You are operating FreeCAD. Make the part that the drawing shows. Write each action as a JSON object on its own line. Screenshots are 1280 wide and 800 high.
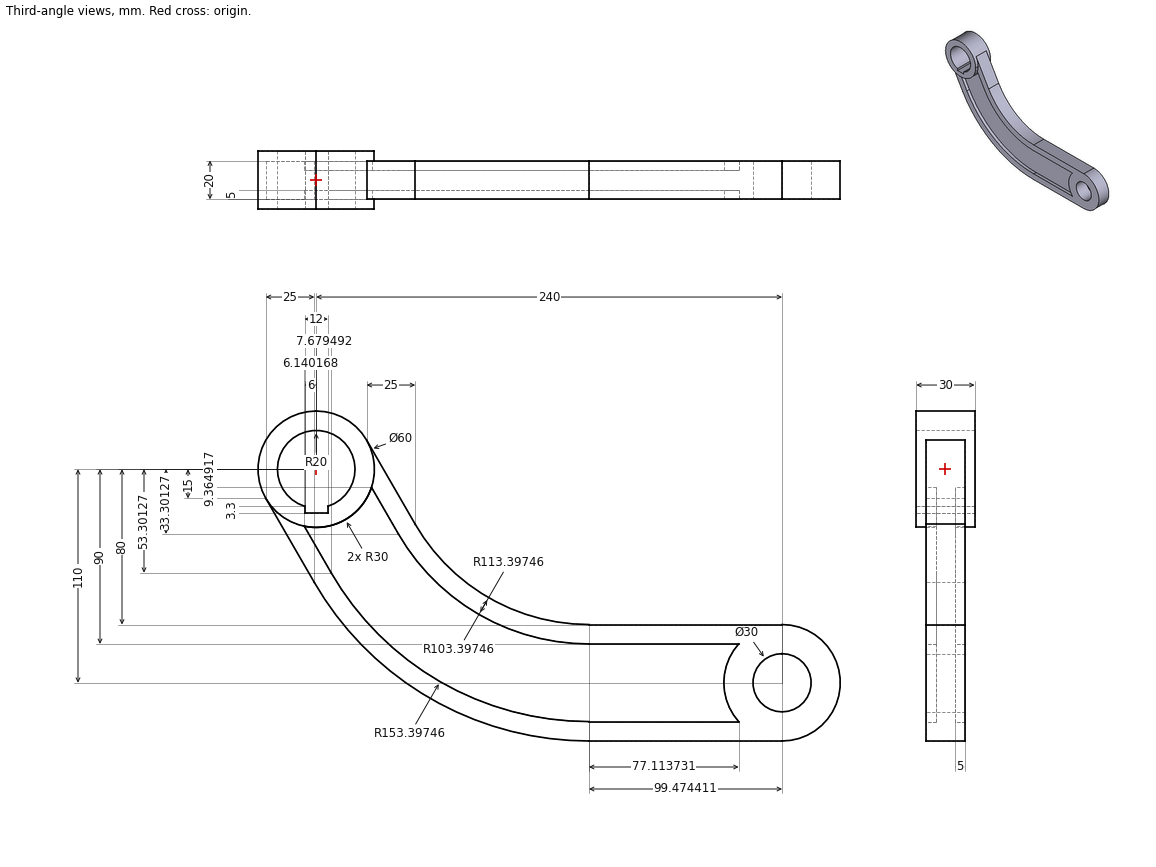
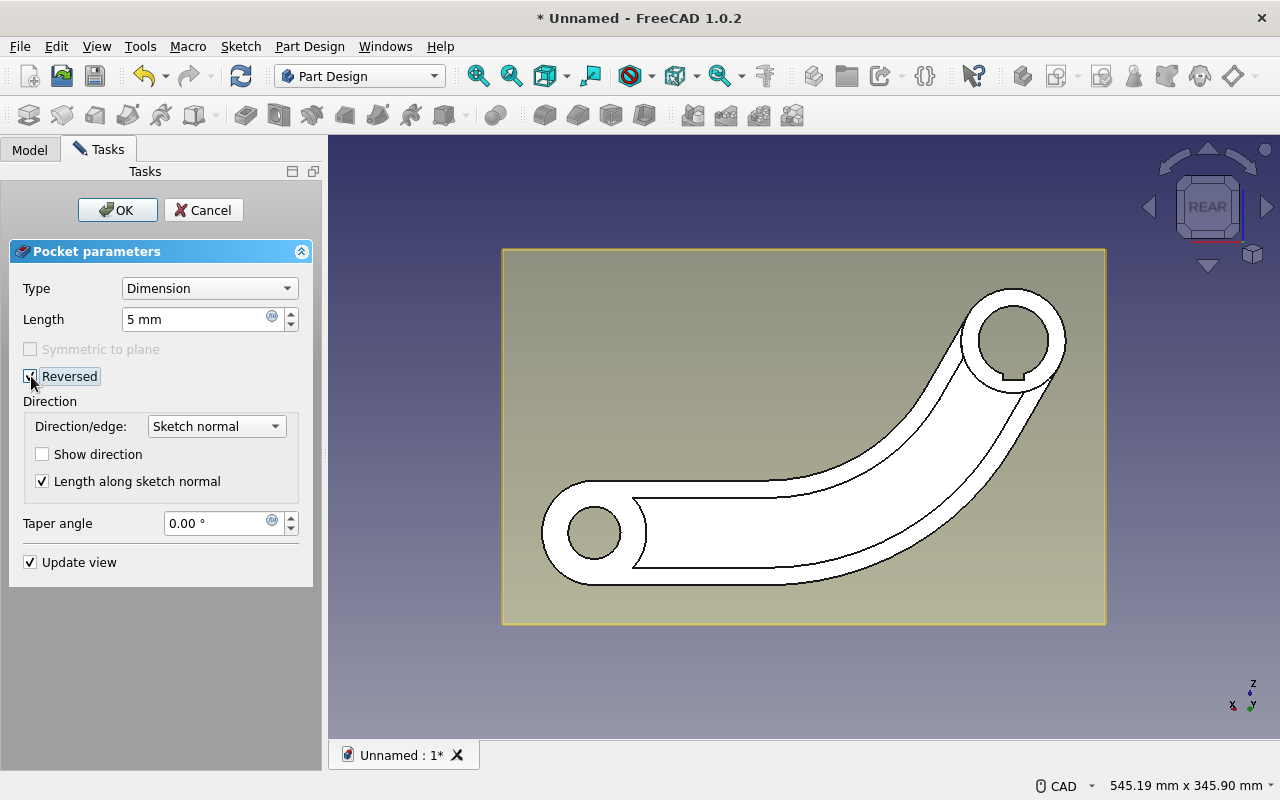
{"action": "left_click", "coordinate": [118, 210]}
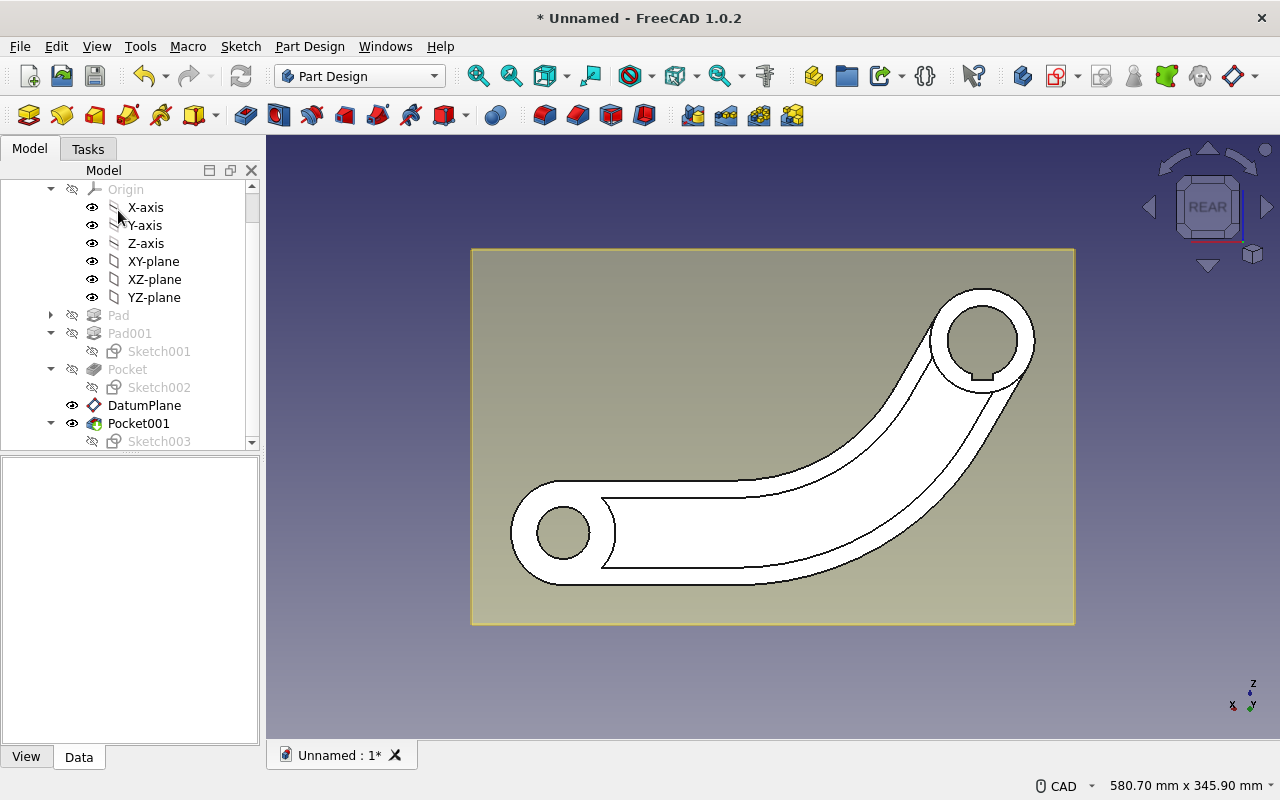
{"action": "left_click", "coordinate": [117, 405]}
{"action": "key", "text": "space"}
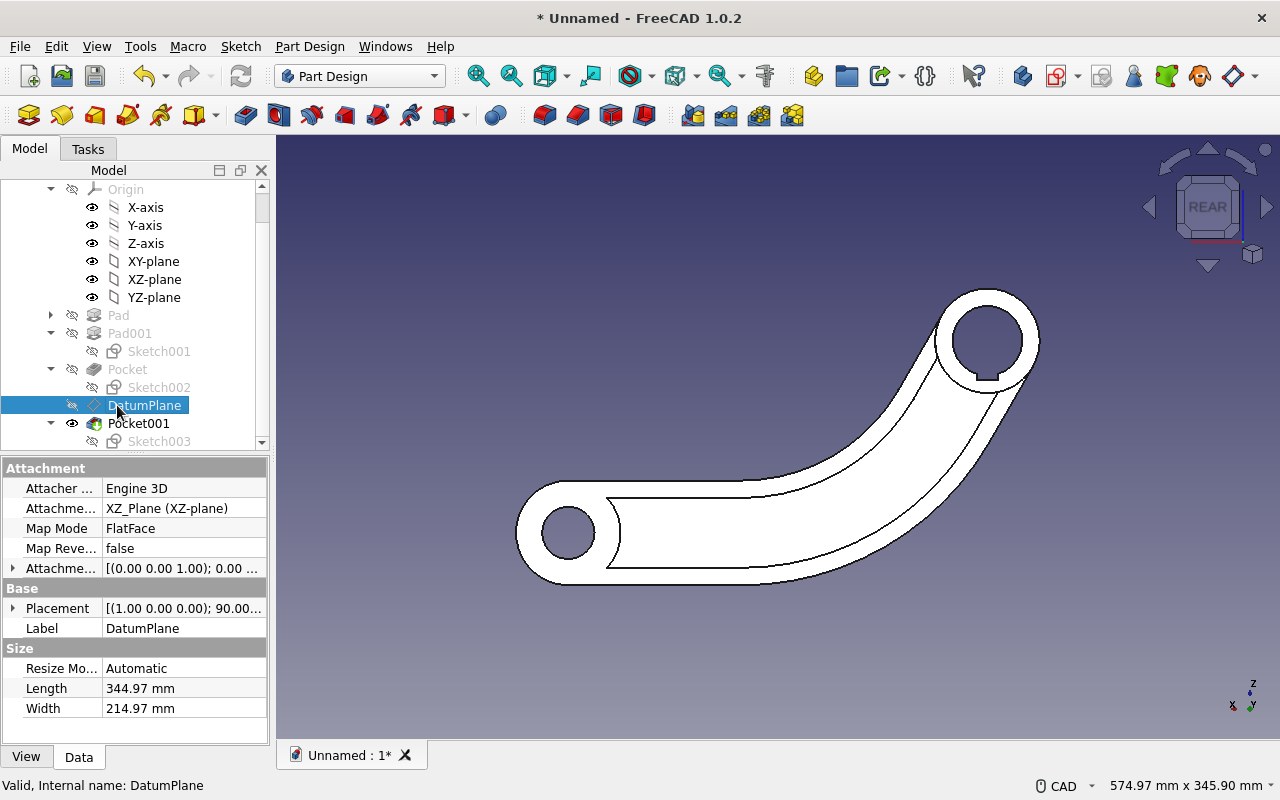
{"action": "key", "text": "0"}